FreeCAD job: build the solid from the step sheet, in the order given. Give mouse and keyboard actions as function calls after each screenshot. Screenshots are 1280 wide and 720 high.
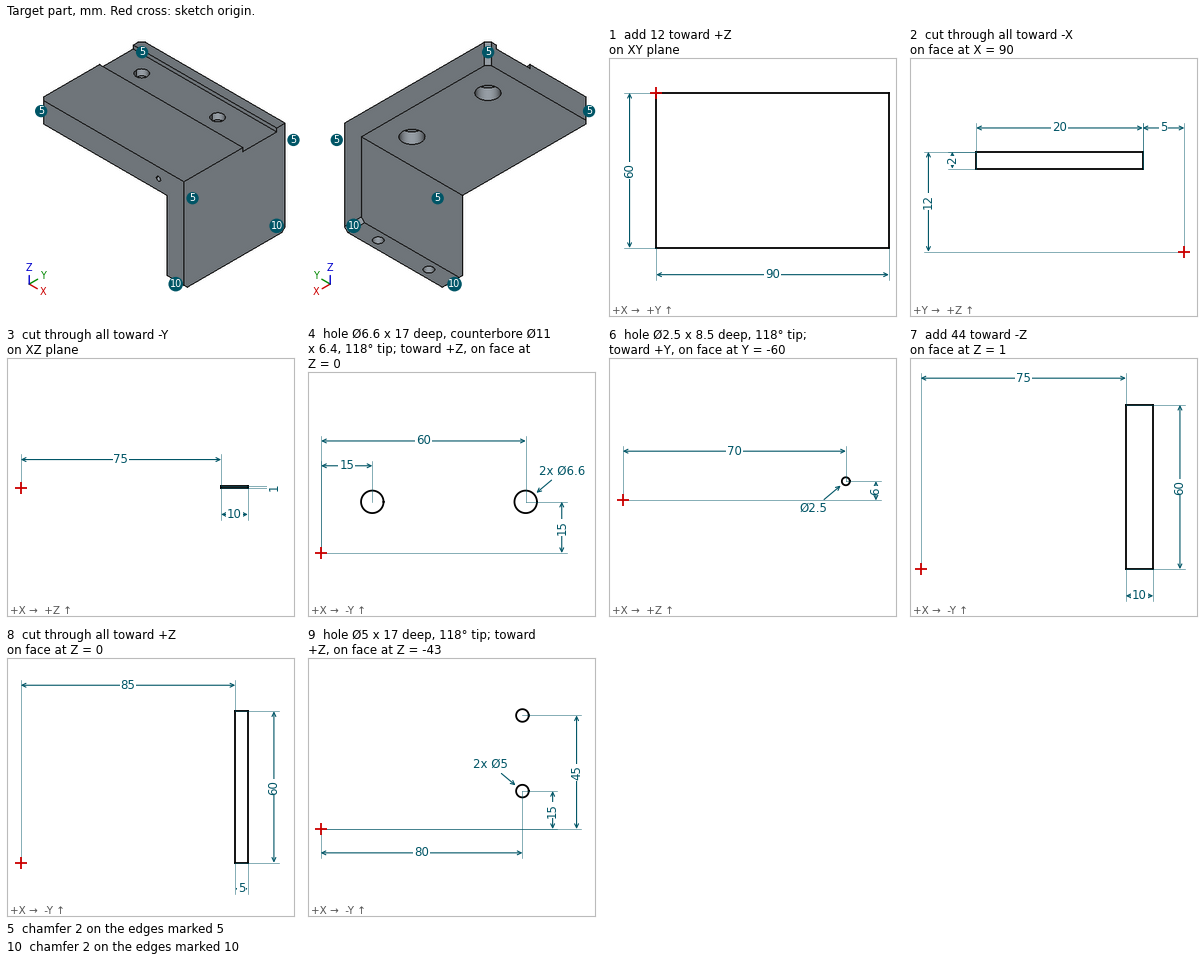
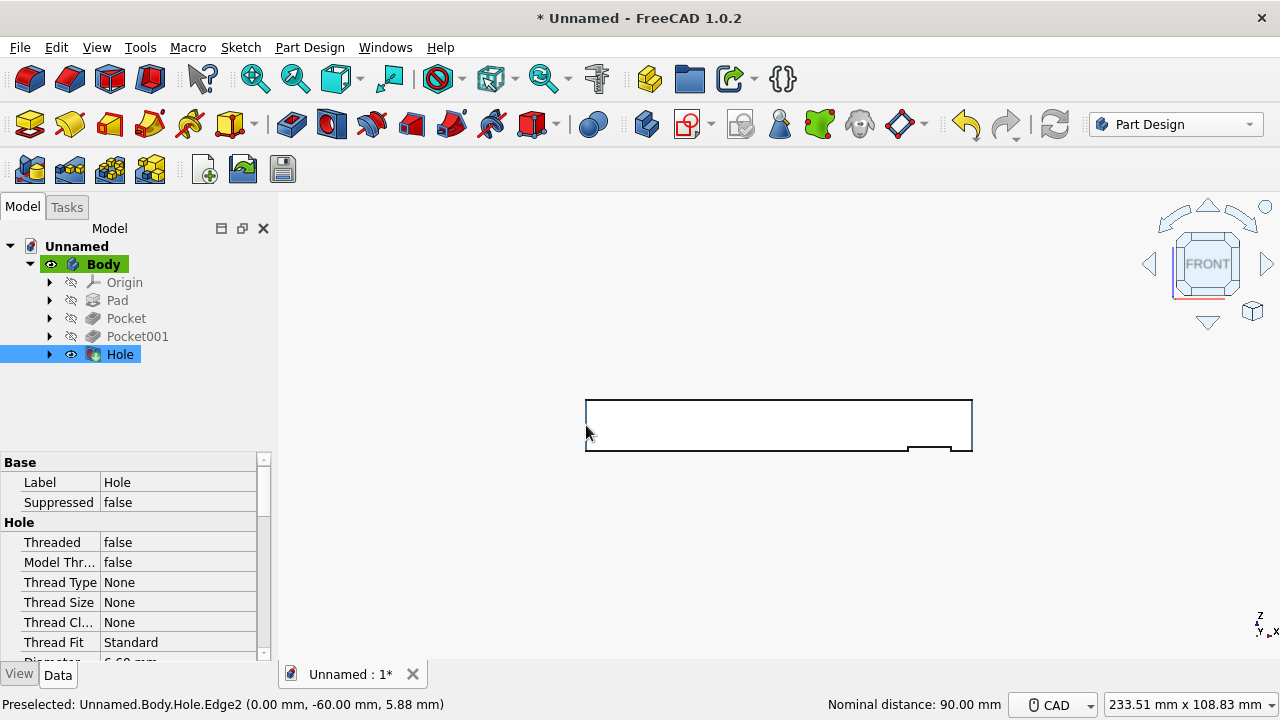
key(3)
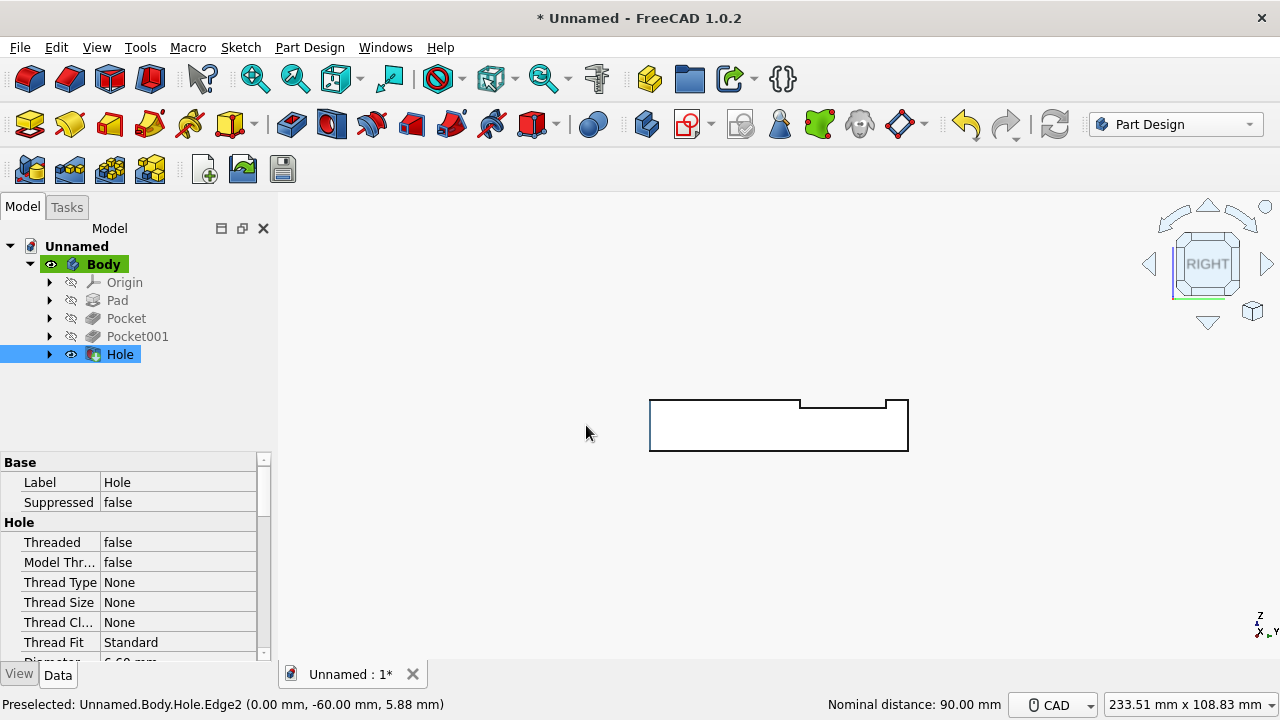
click(256, 80)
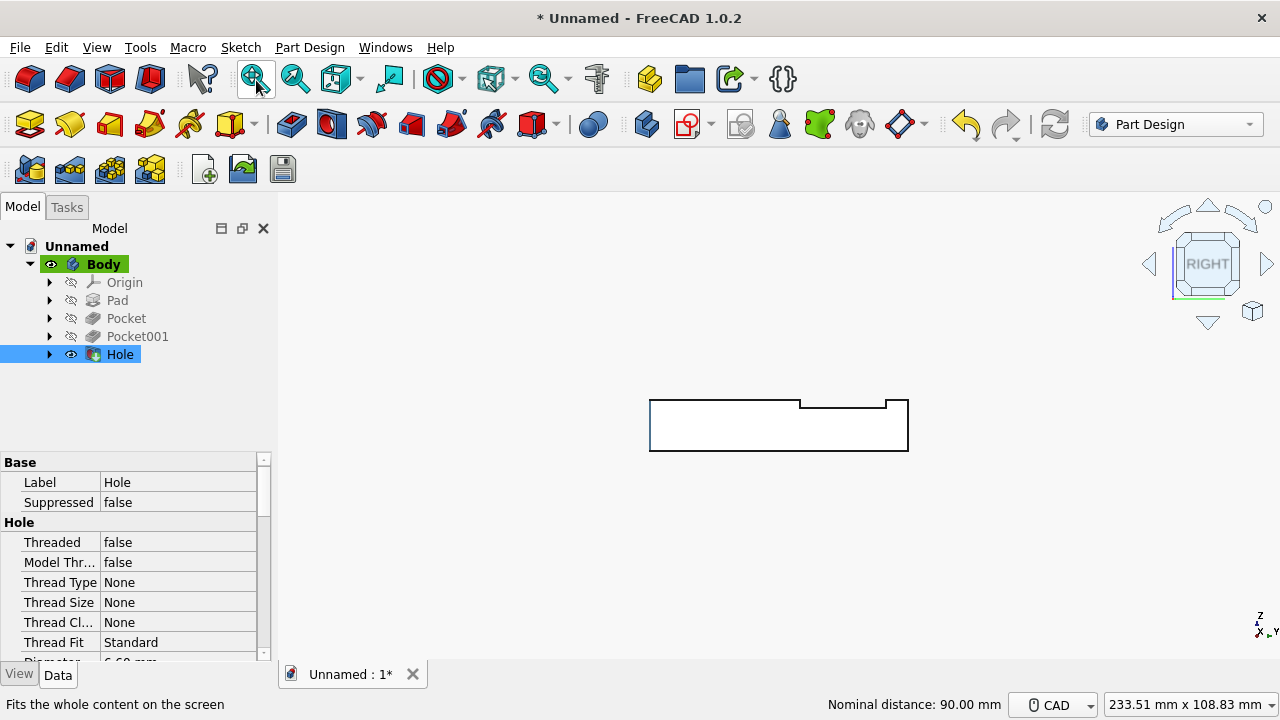
click(908, 424, ctrl)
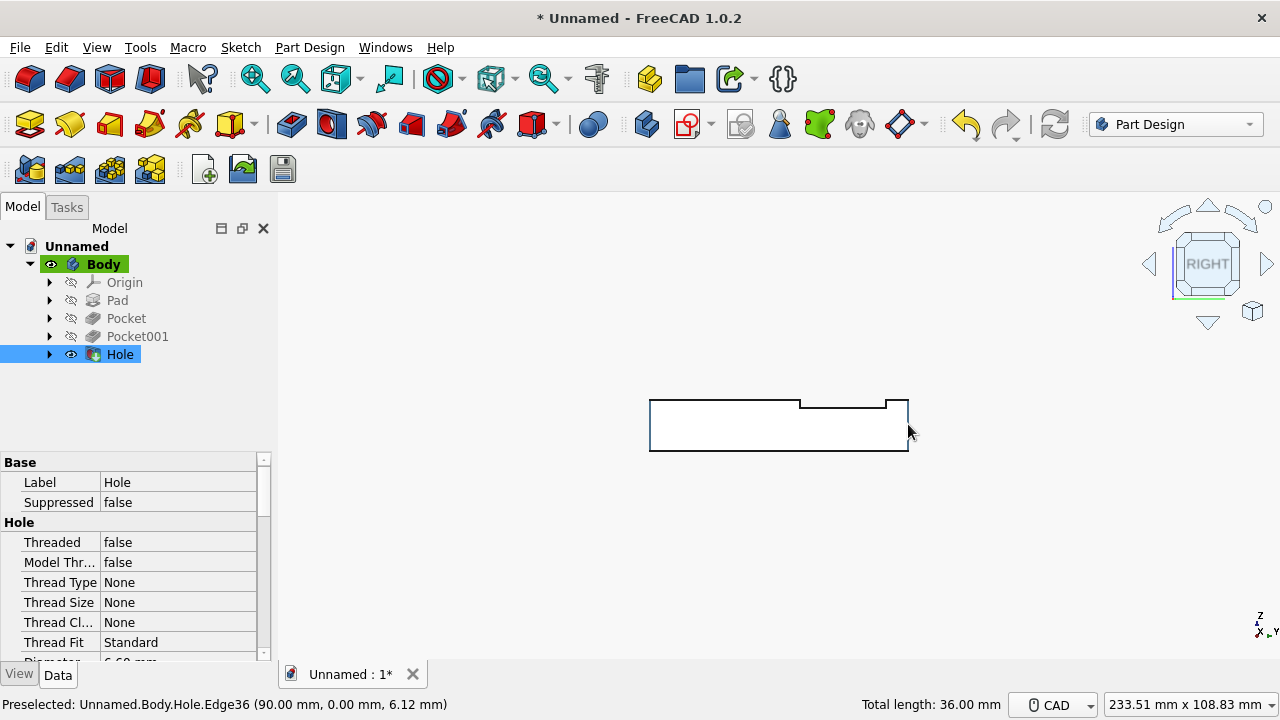
key(5)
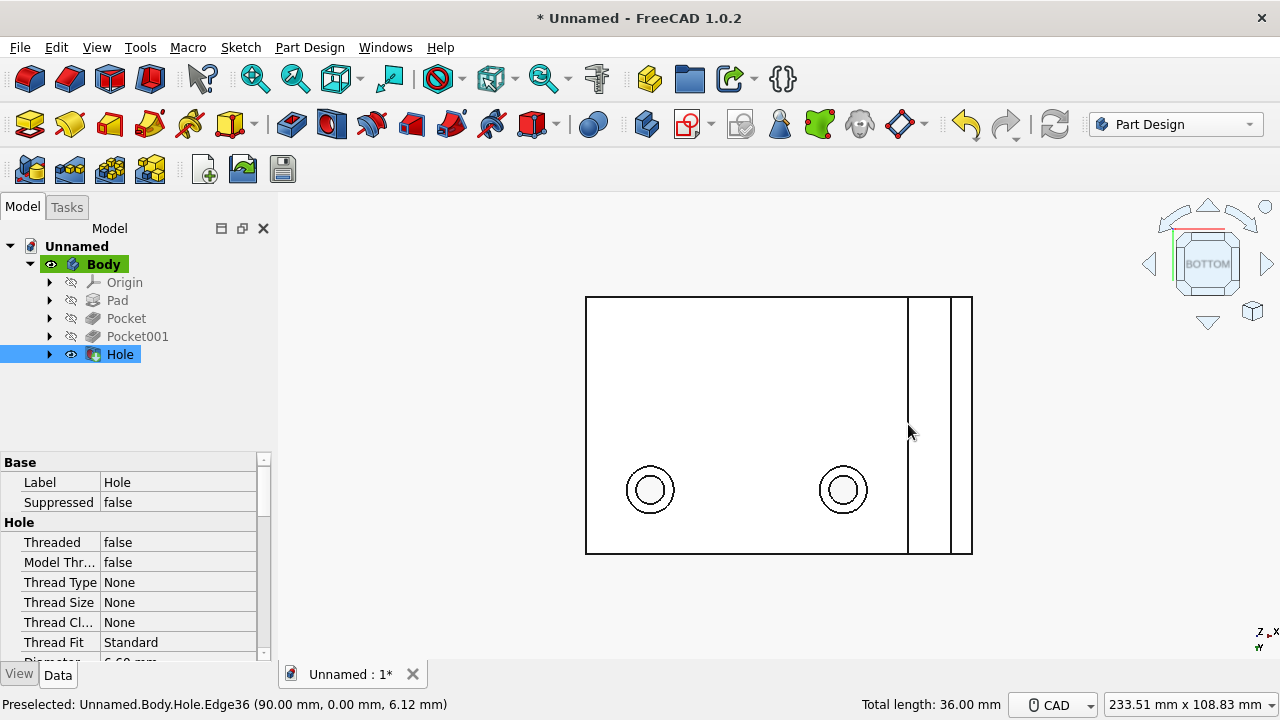
key(4)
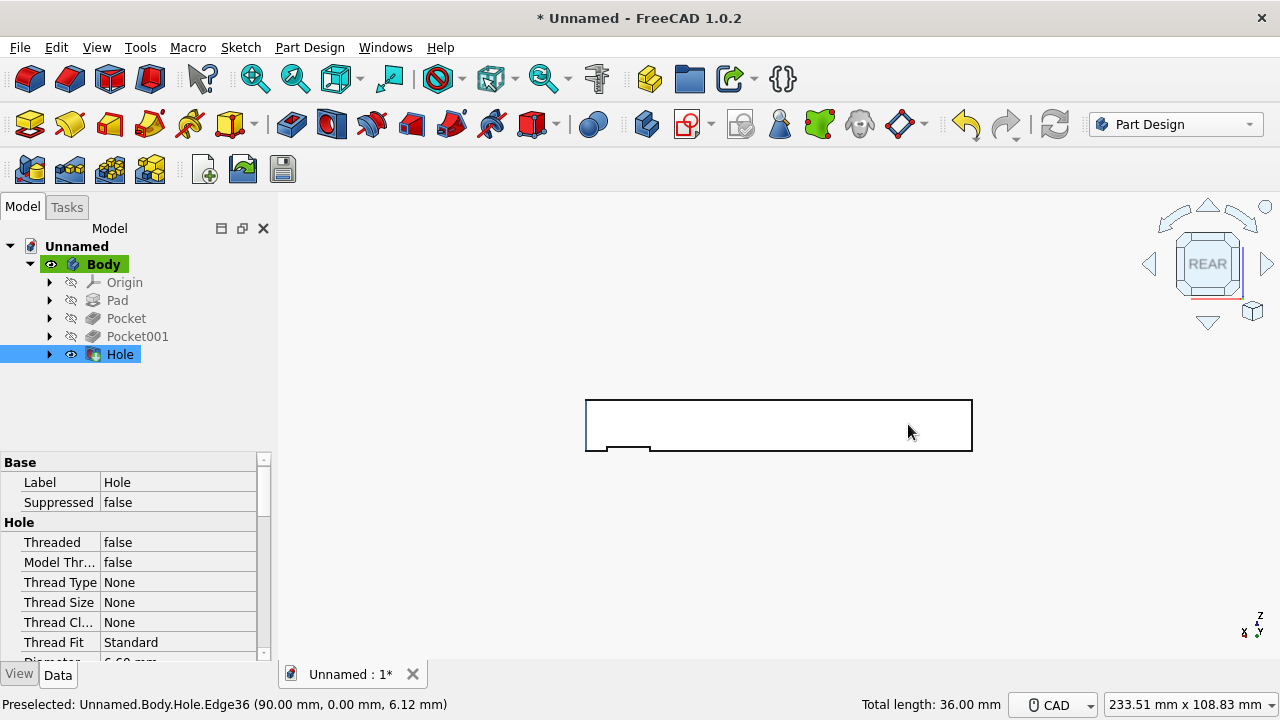
click(256, 80)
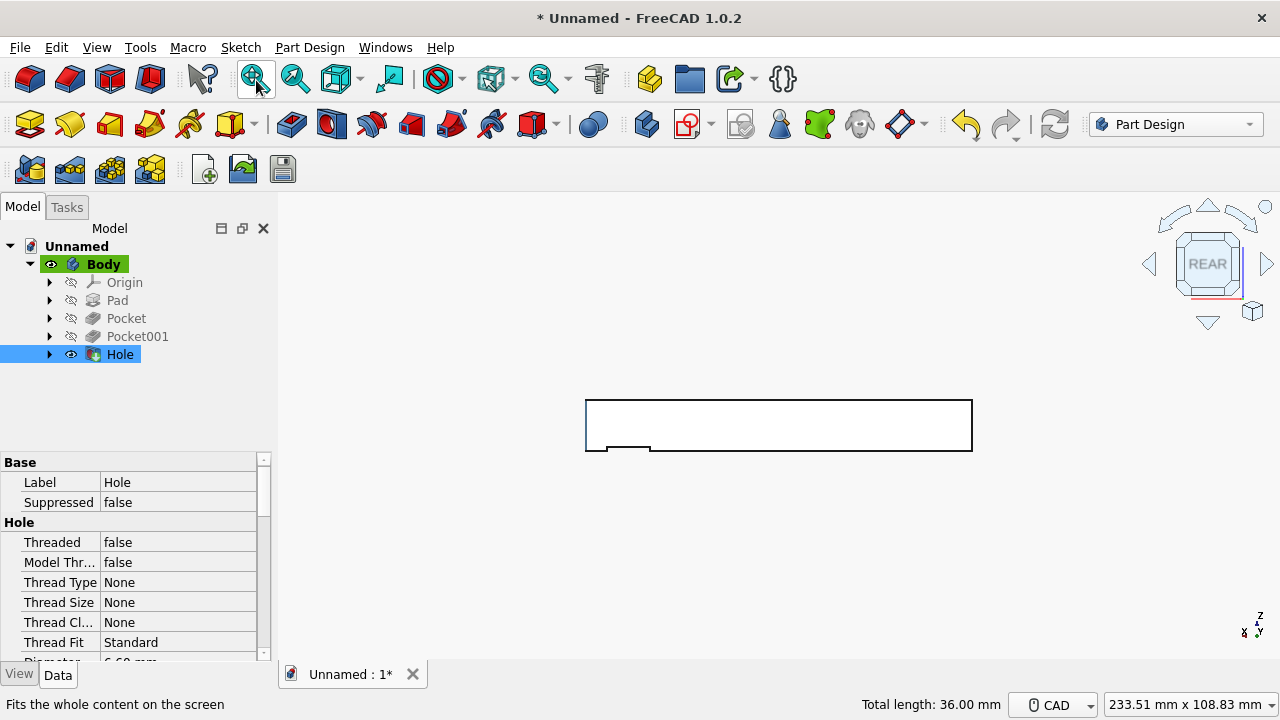
click(972, 425, ctrl)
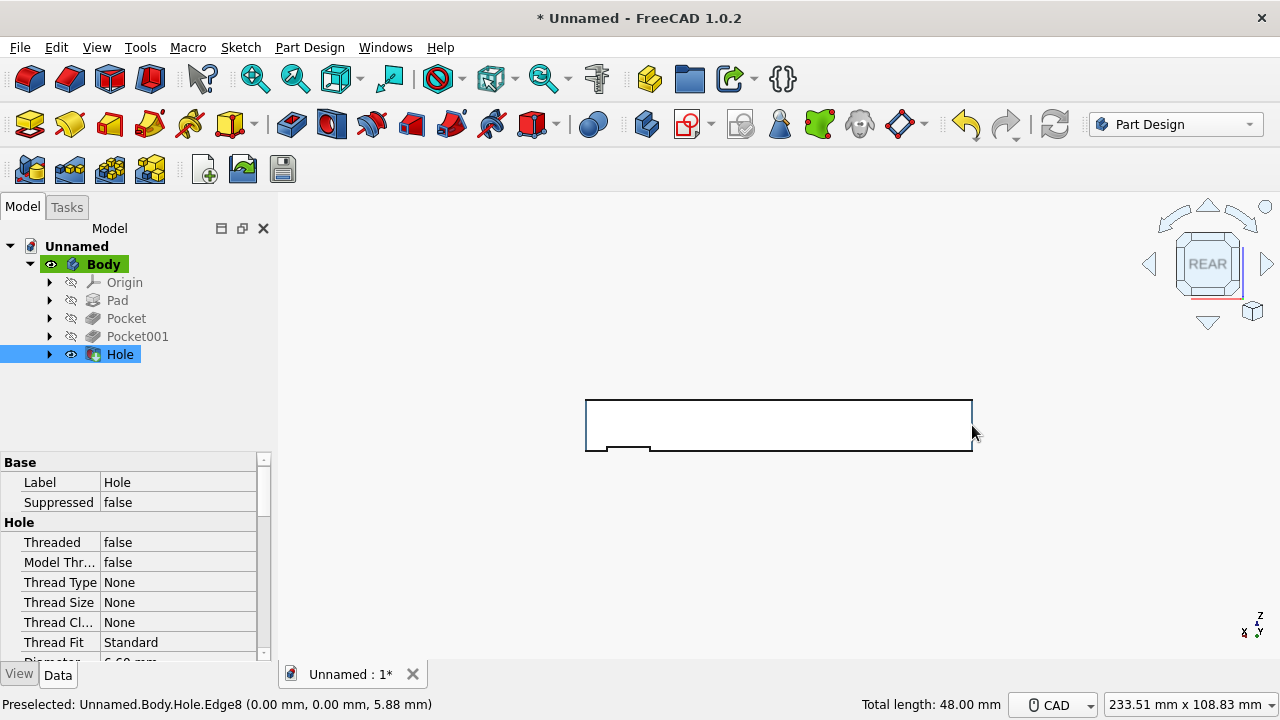
click(70, 80)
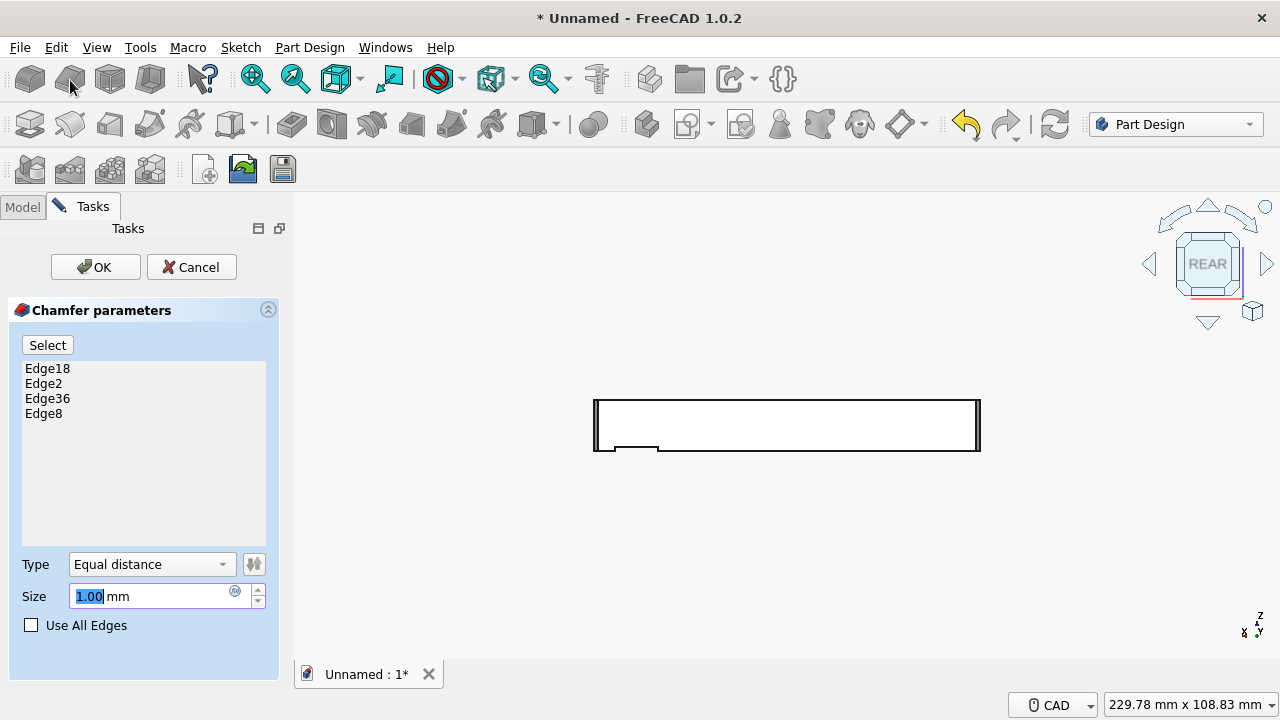
text(2)
key(Tab)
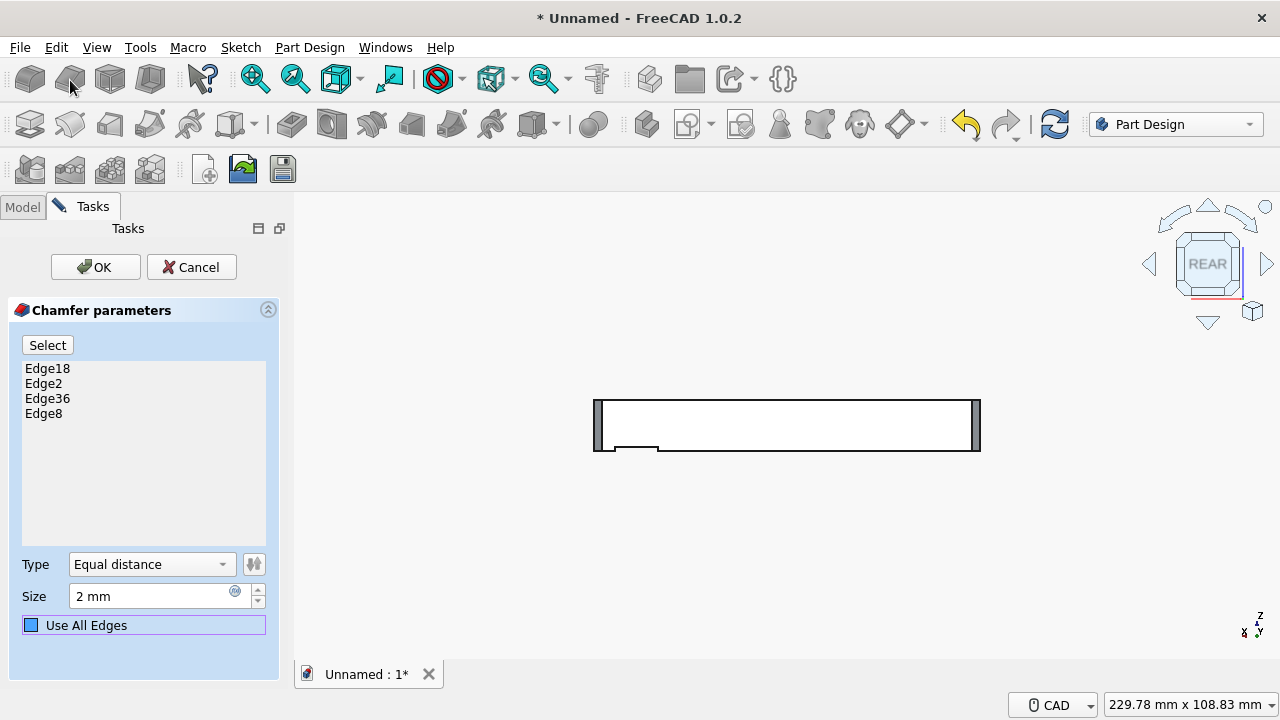
click(96, 267)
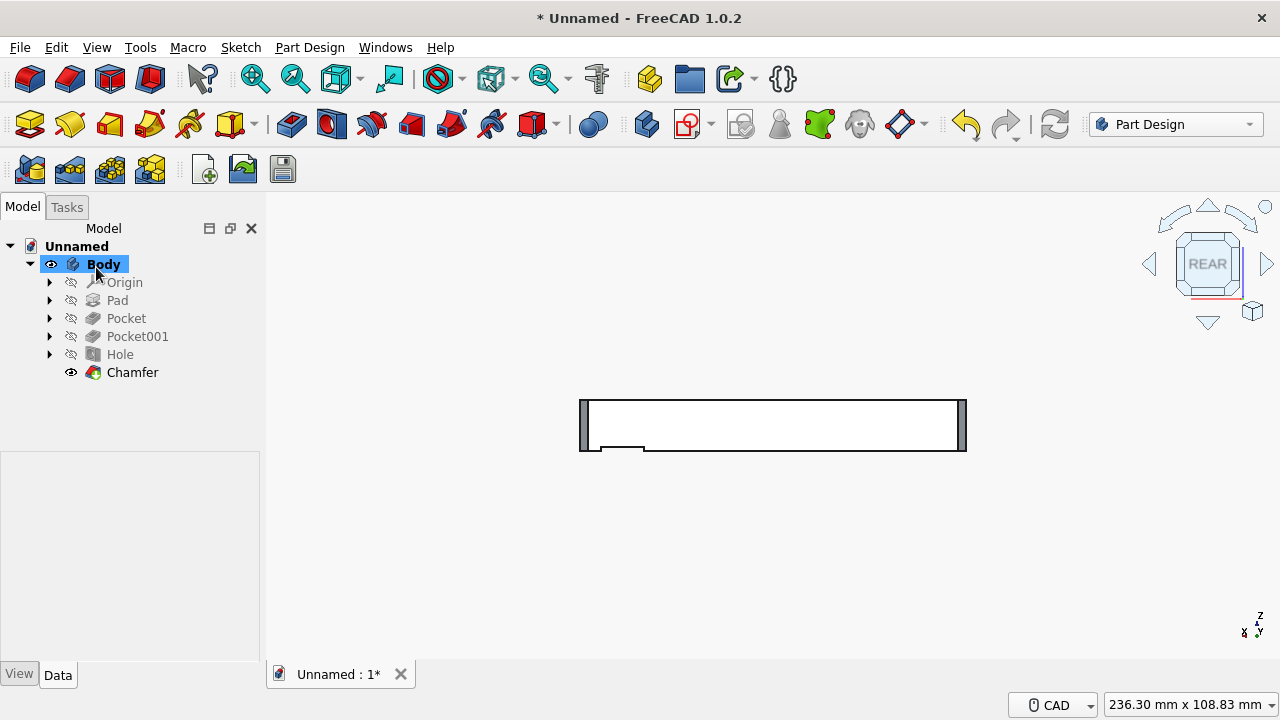
click(256, 80)